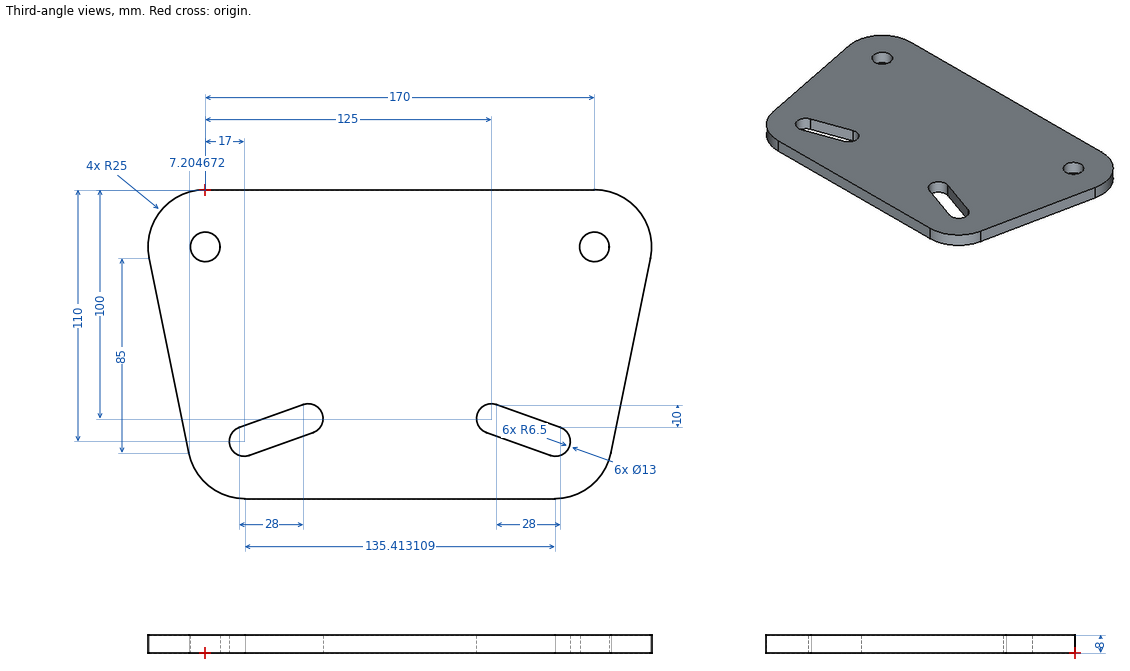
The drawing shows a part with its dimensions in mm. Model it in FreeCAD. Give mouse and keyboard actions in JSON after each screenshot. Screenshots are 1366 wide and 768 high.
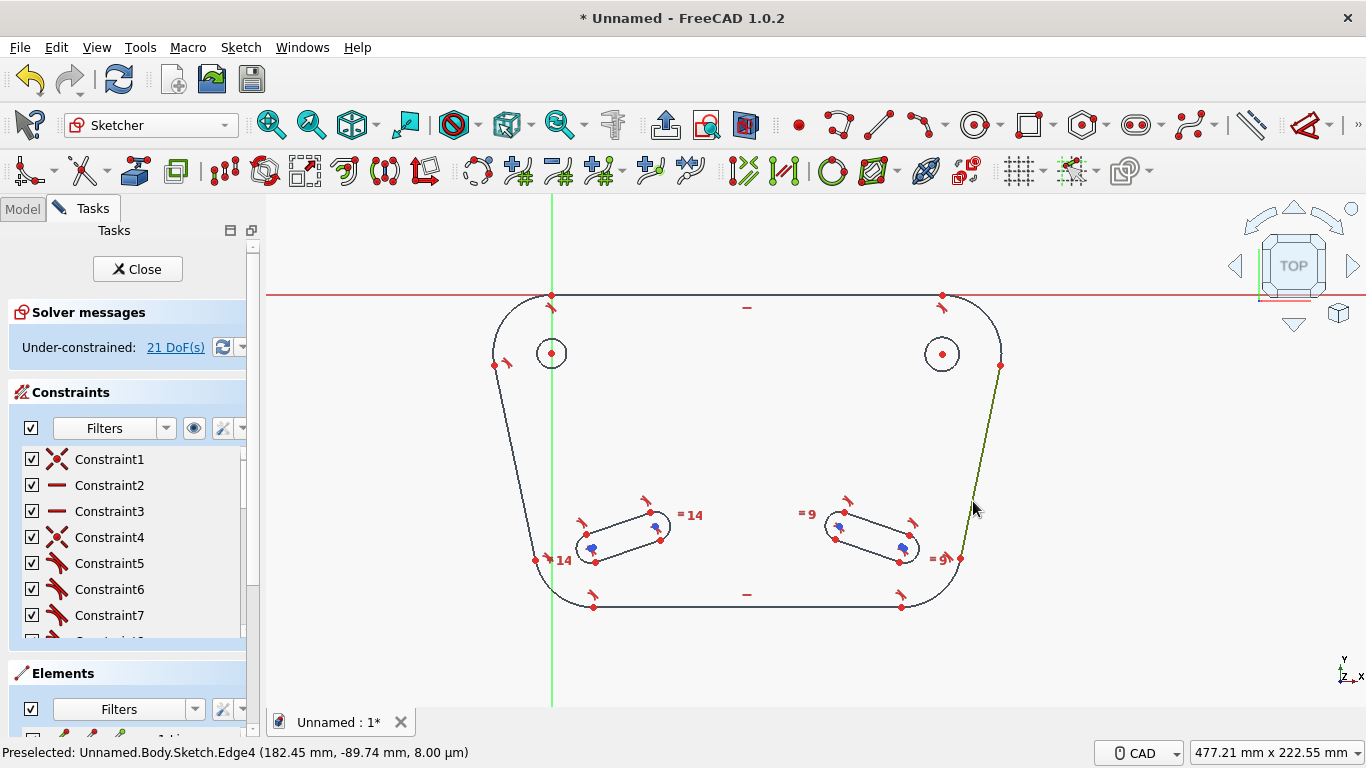
{"action": "left_click", "coordinate": [998, 335]}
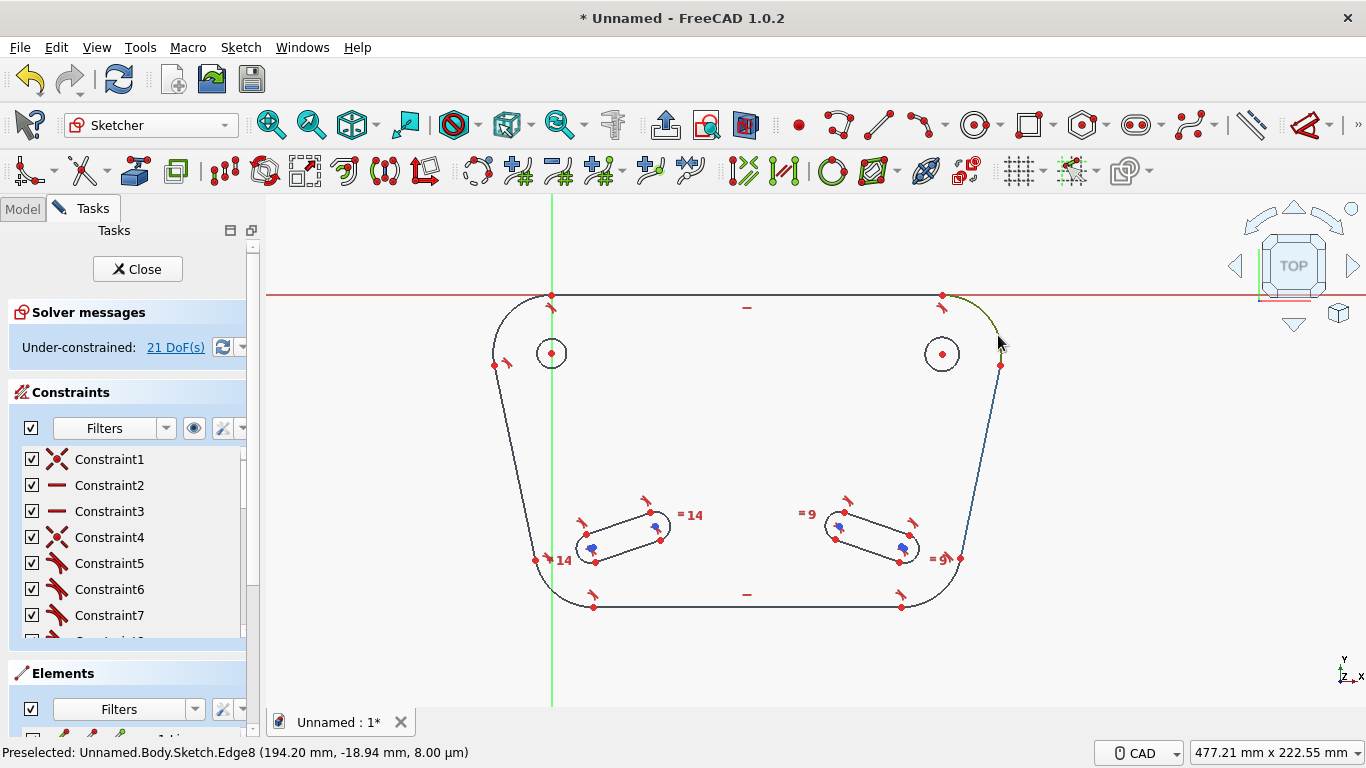
{"action": "key", "text": "t"}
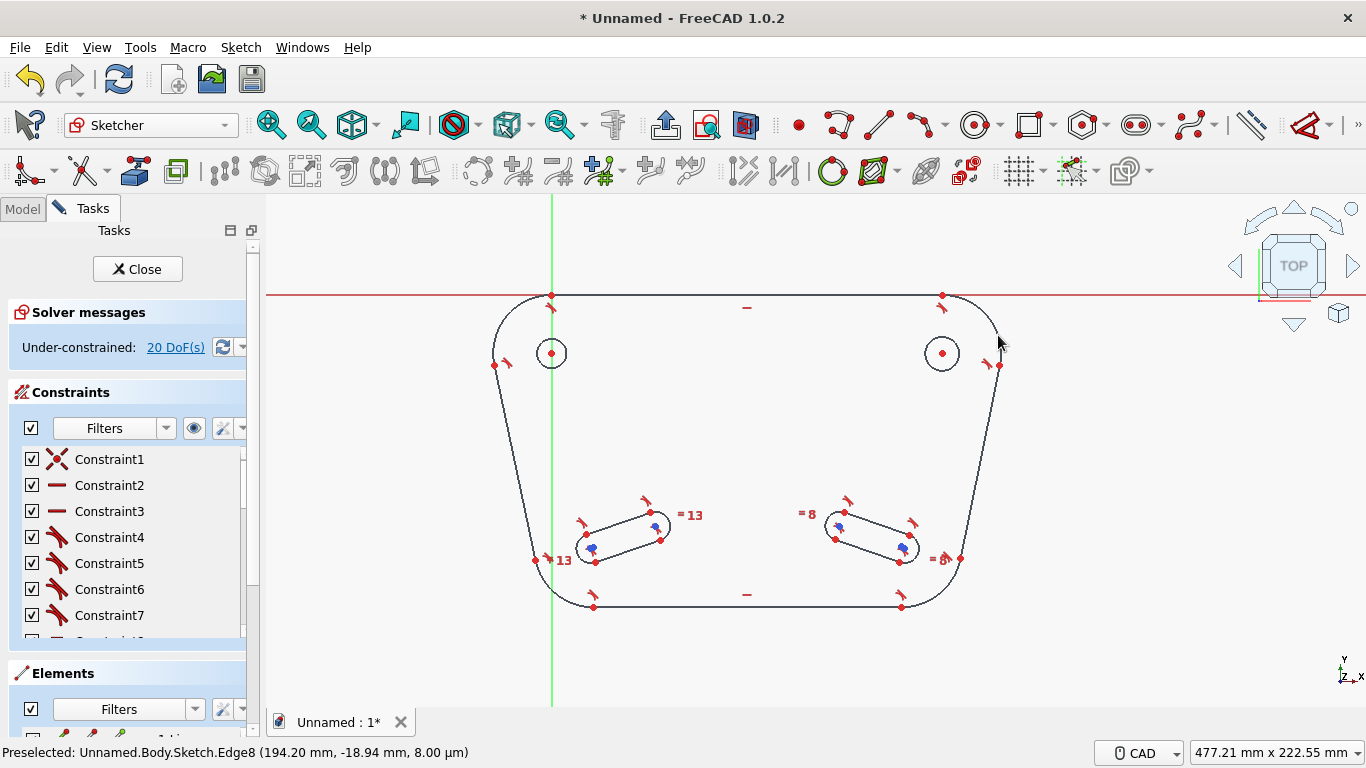
{"action": "left_click", "coordinate": [496, 335]}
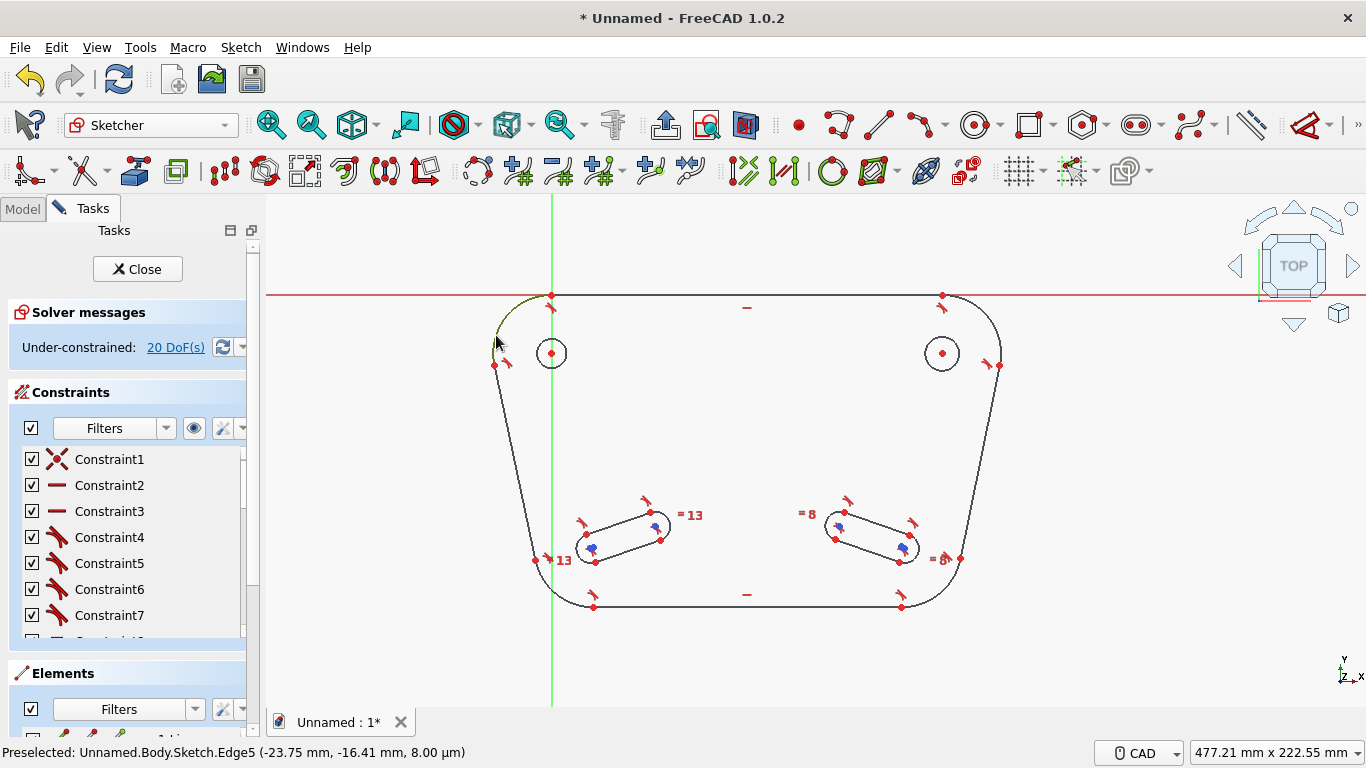
{"action": "left_click", "coordinate": [570, 602]}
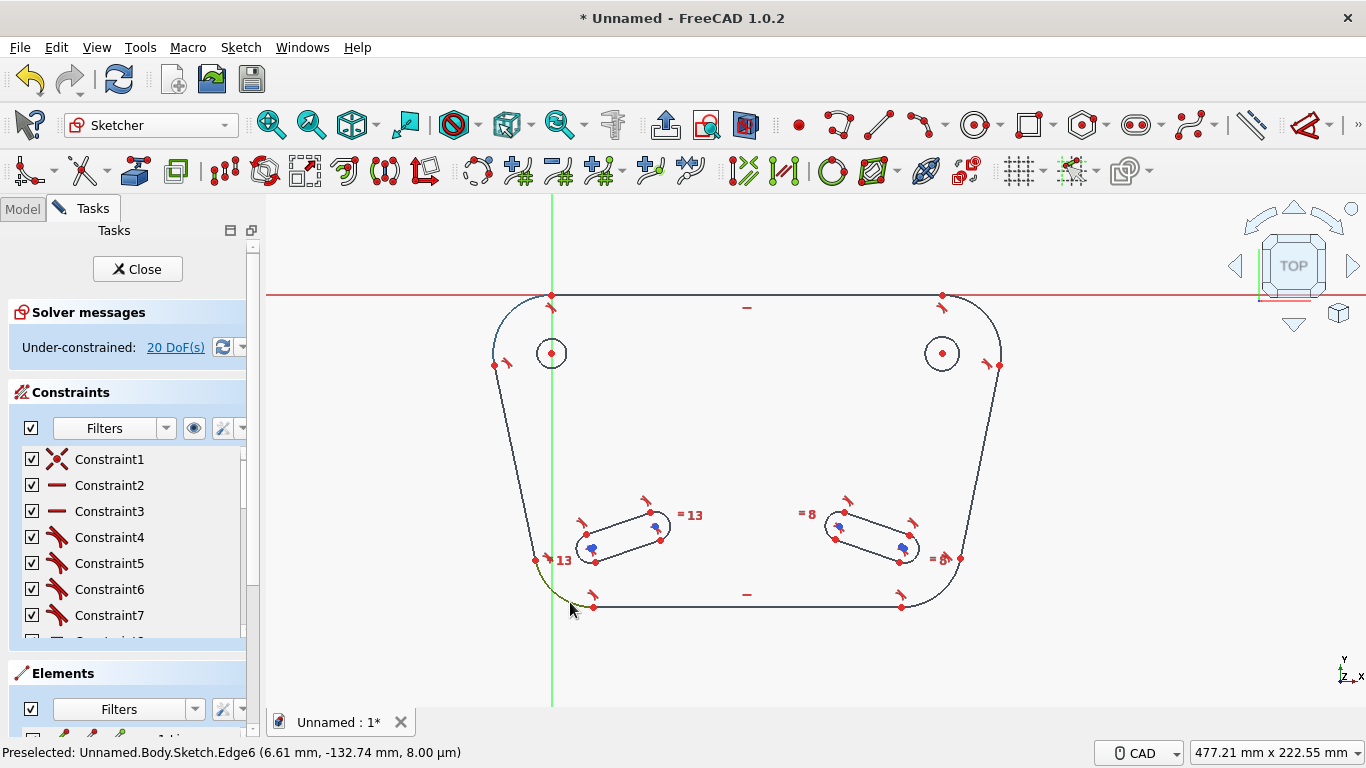
{"action": "left_click", "coordinate": [925, 602]}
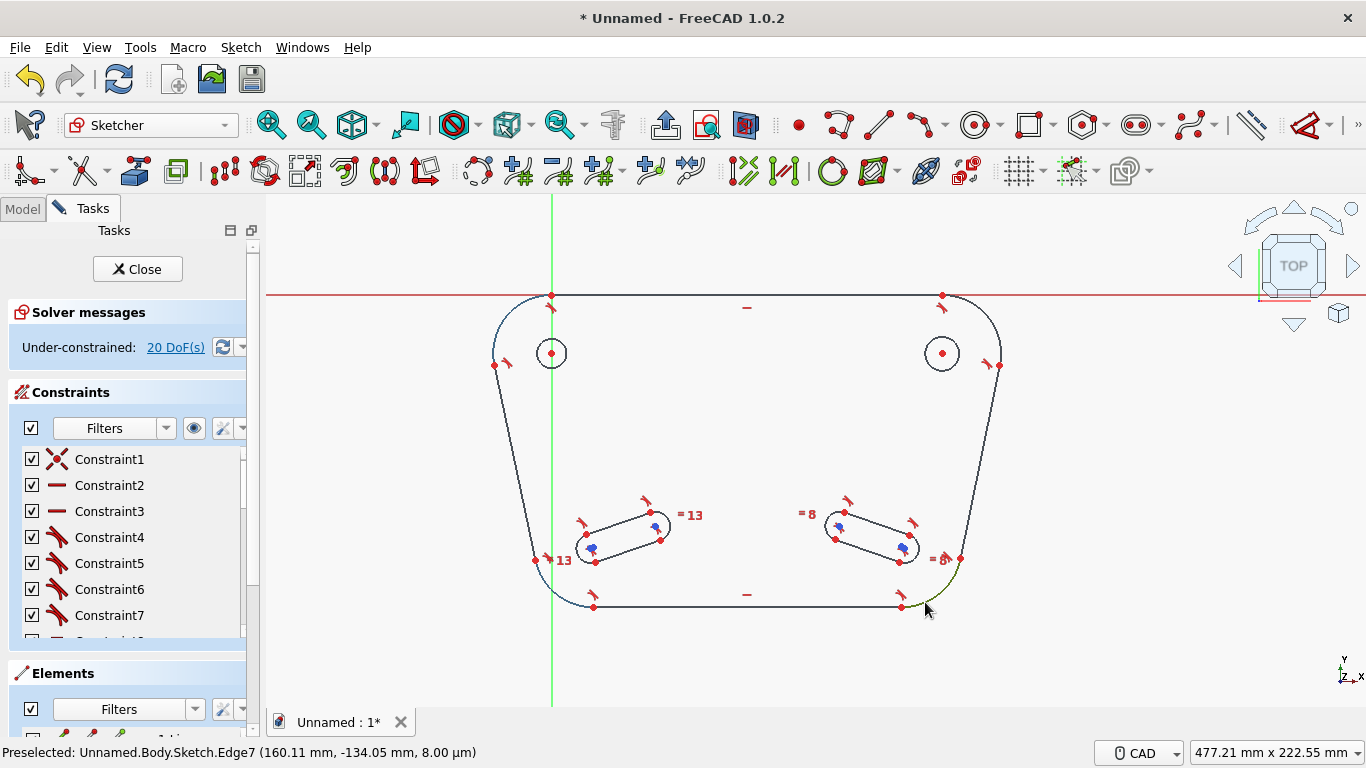
{"action": "left_click", "coordinate": [998, 335]}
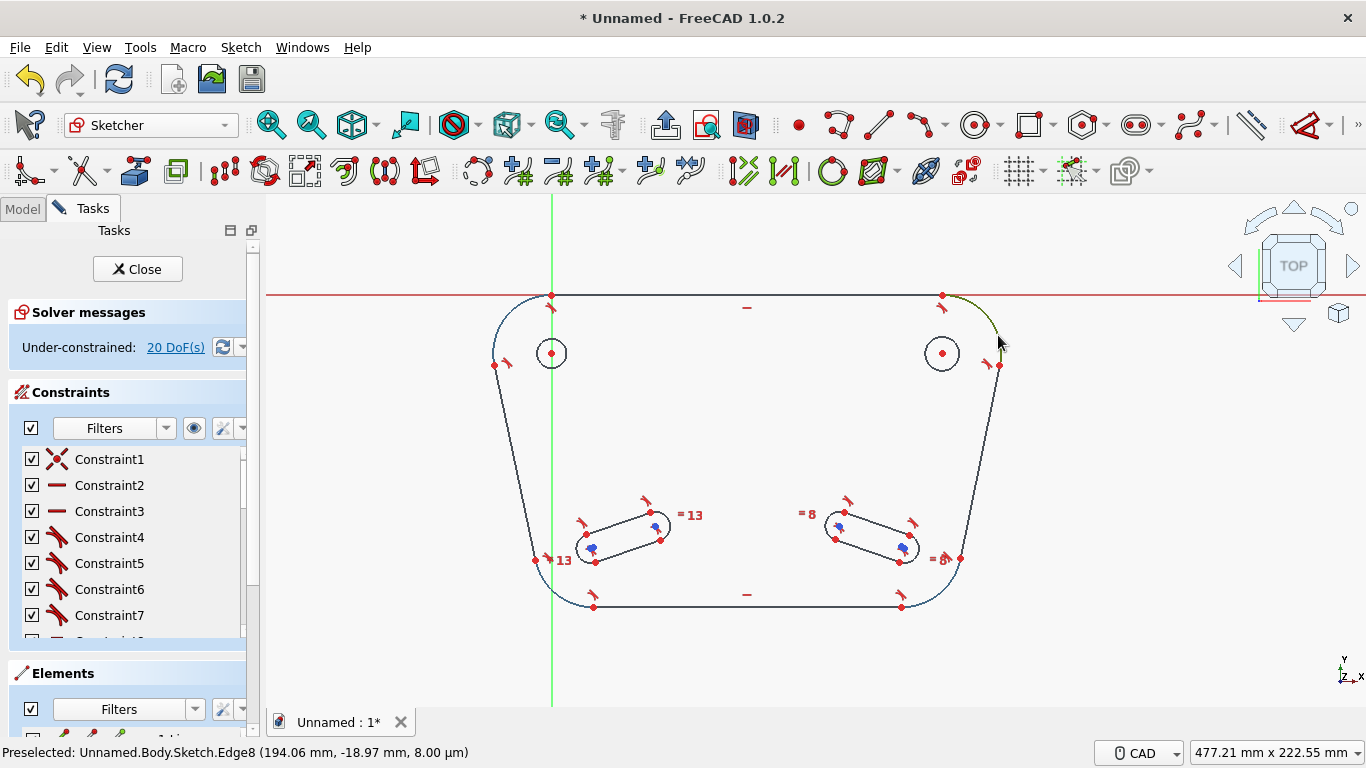
{"action": "key", "text": "e"}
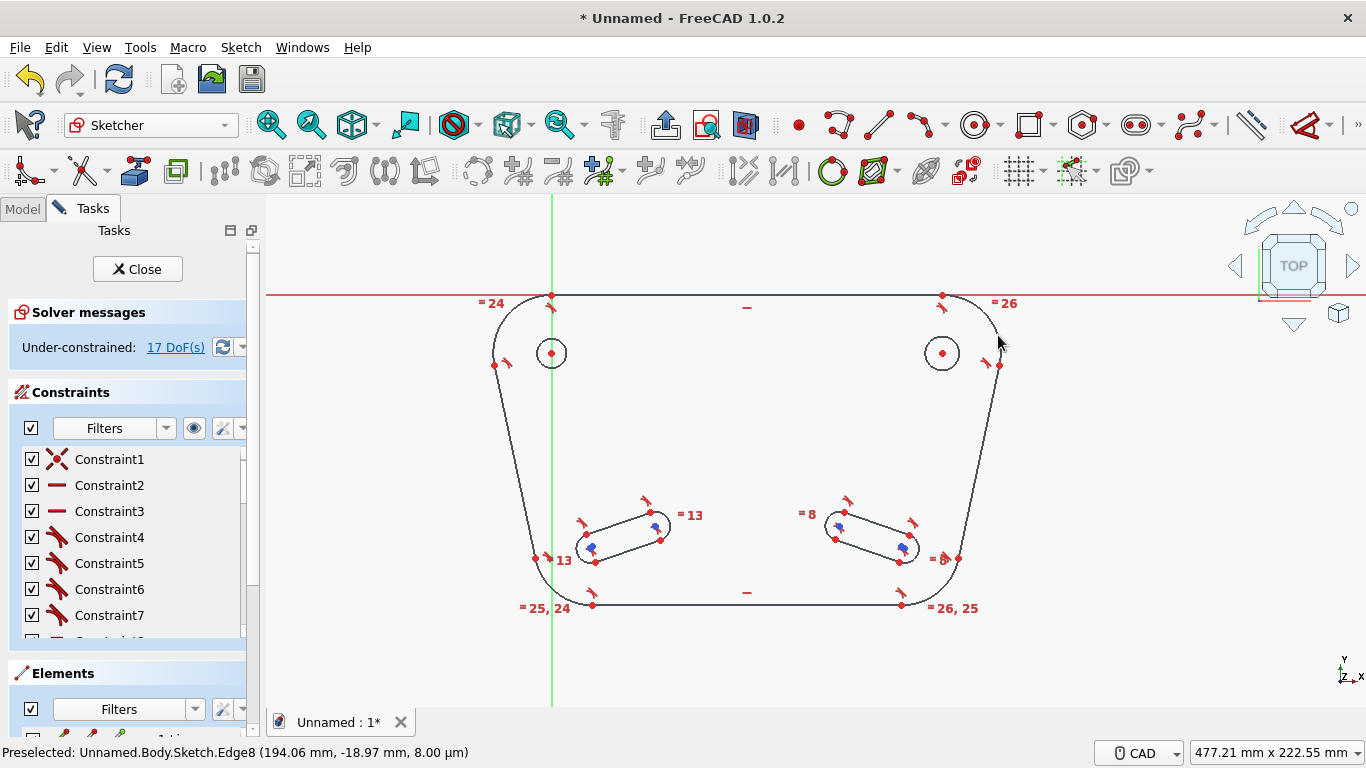
{"action": "left_click", "coordinate": [832, 514]}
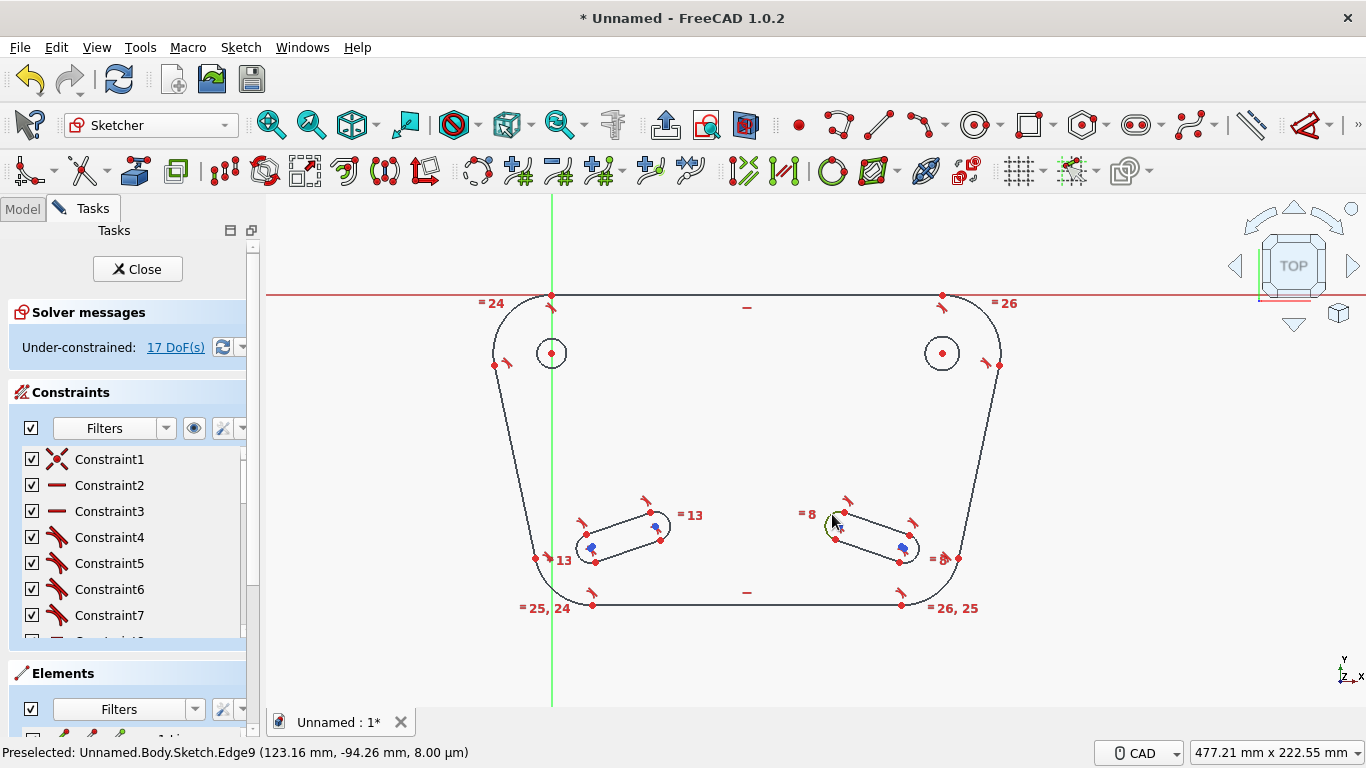
{"action": "left_click", "coordinate": [577, 544]}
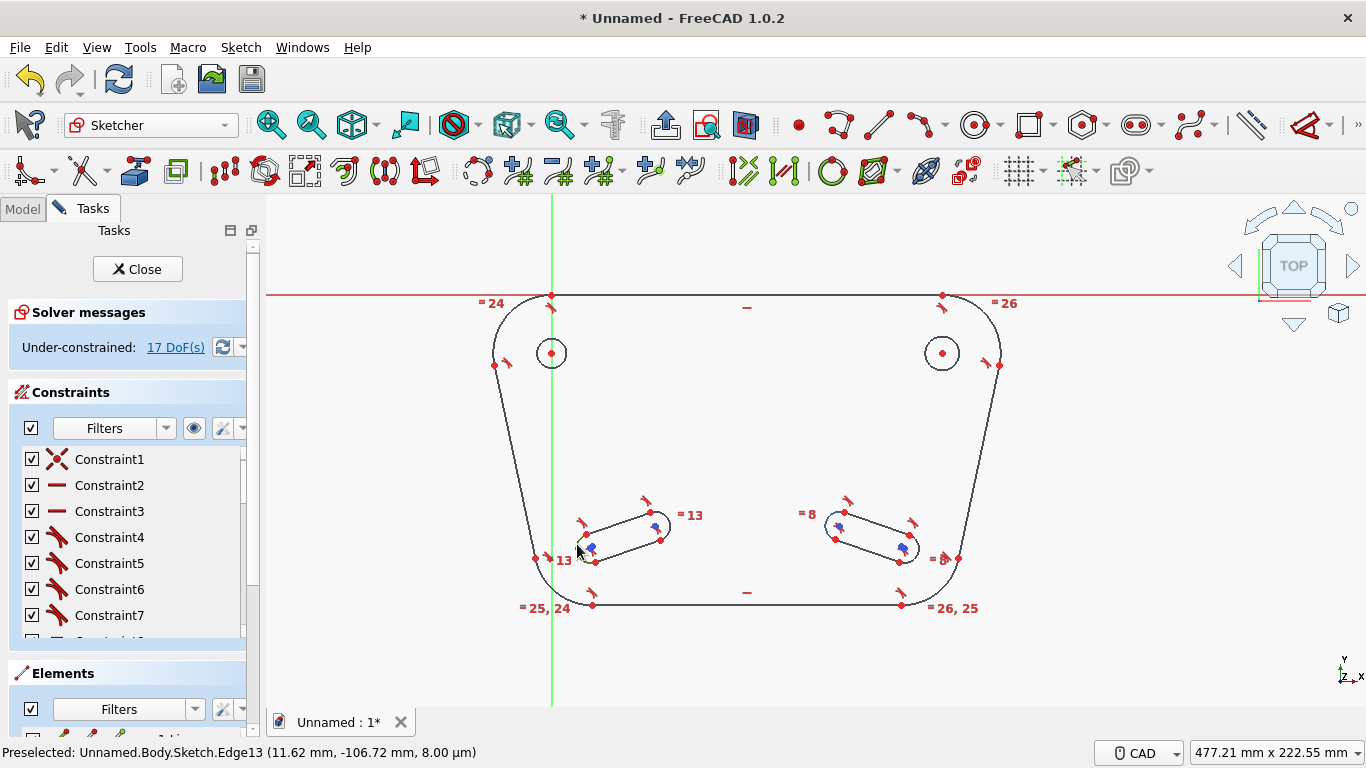
{"action": "key", "text": "e"}